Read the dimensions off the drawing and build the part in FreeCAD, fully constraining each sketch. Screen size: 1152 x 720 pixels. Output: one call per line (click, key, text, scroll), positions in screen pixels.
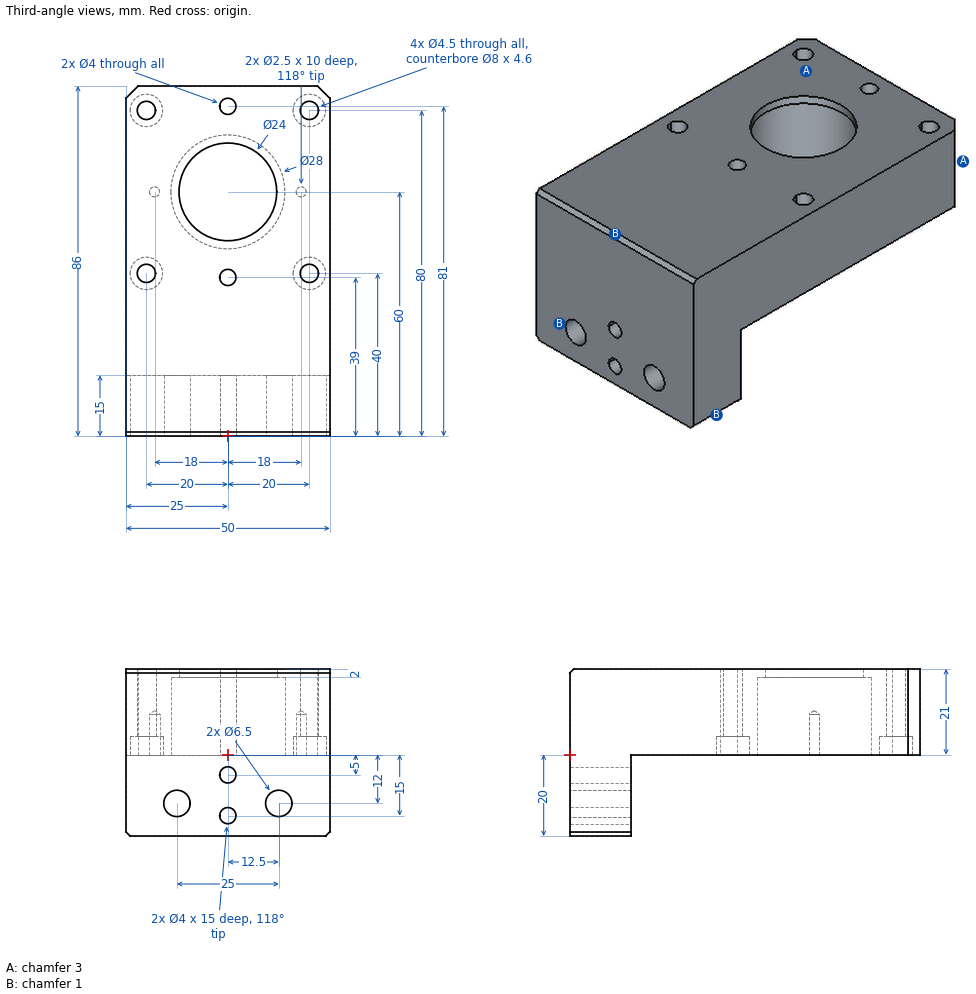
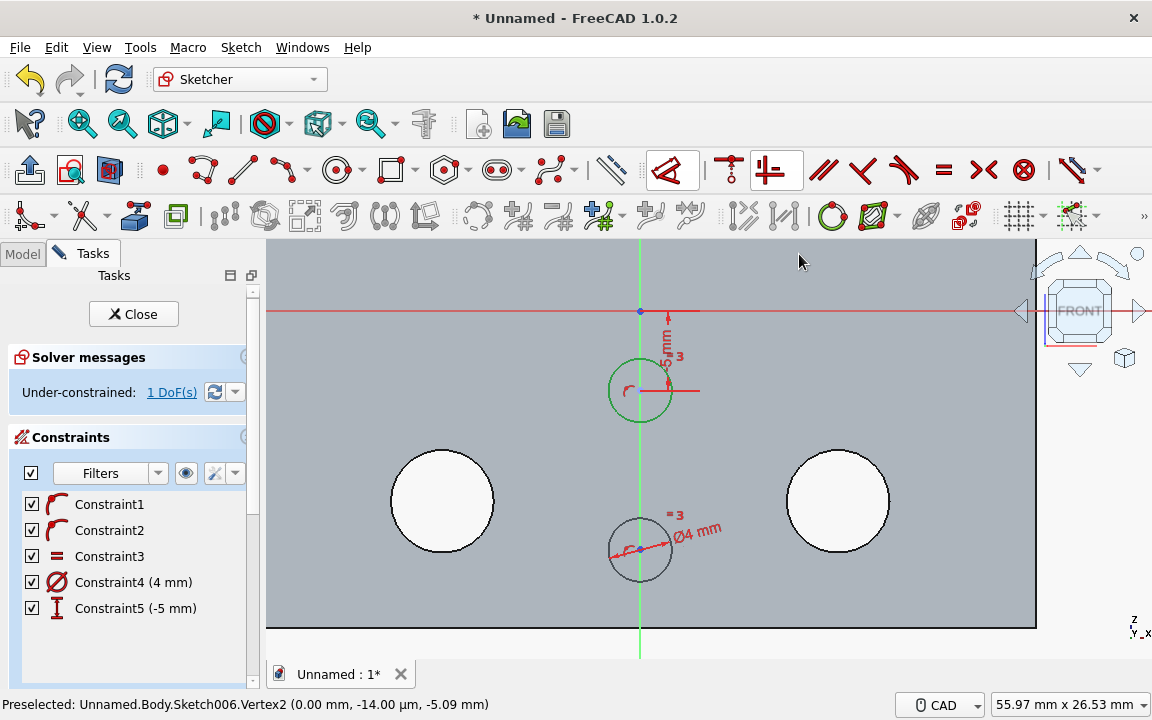
click(640, 550)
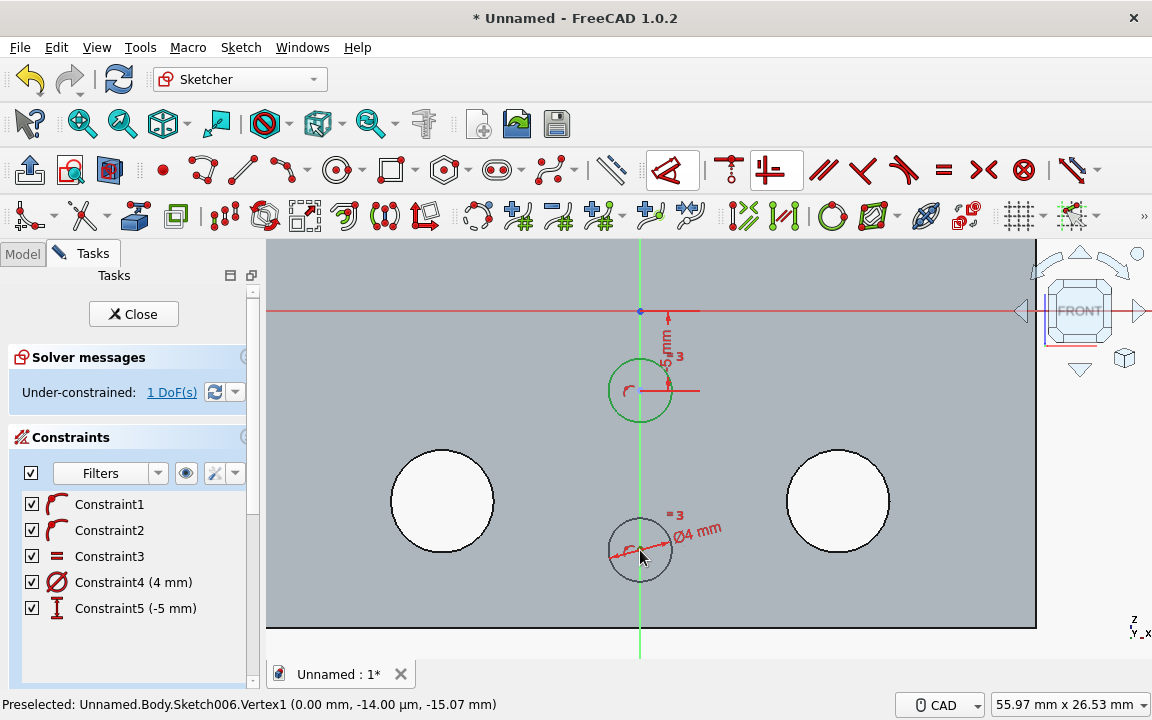
key(i)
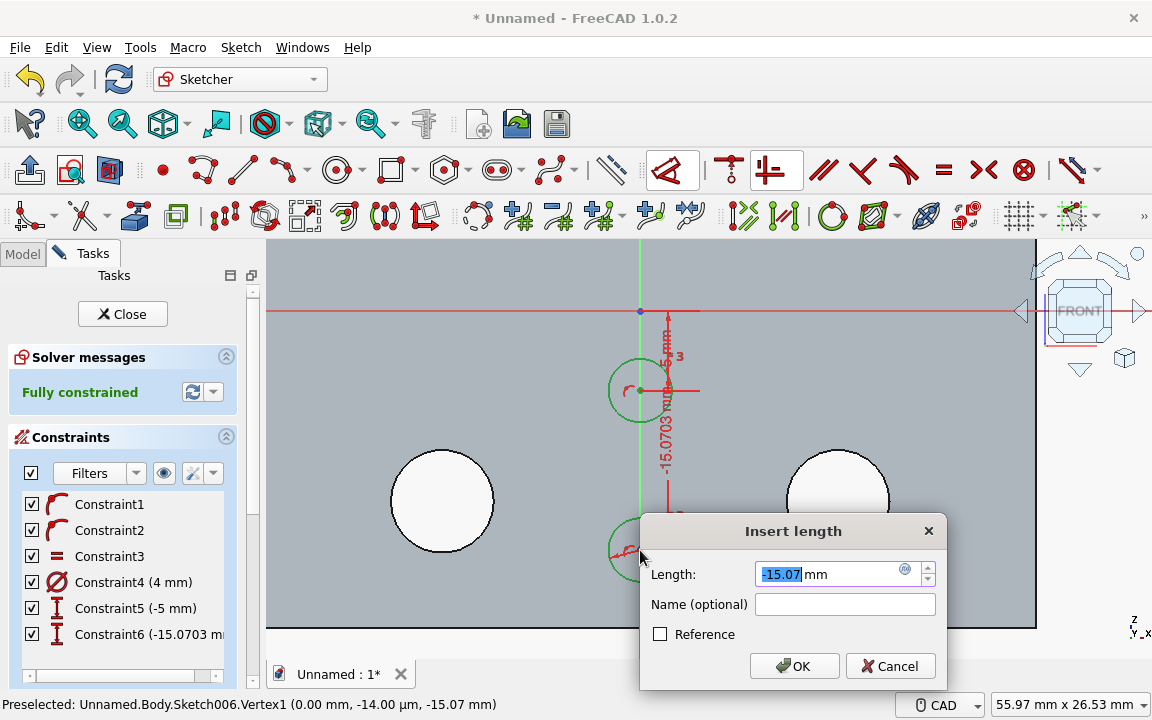
text(-15)
key(Return)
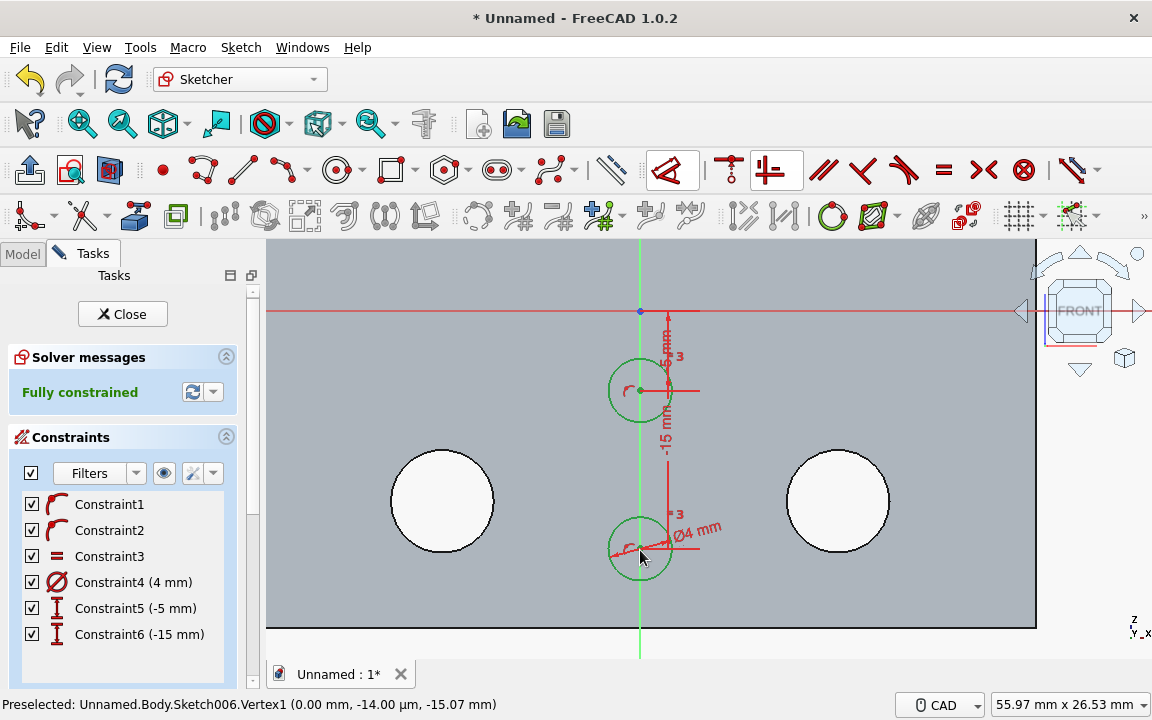
click(123, 314)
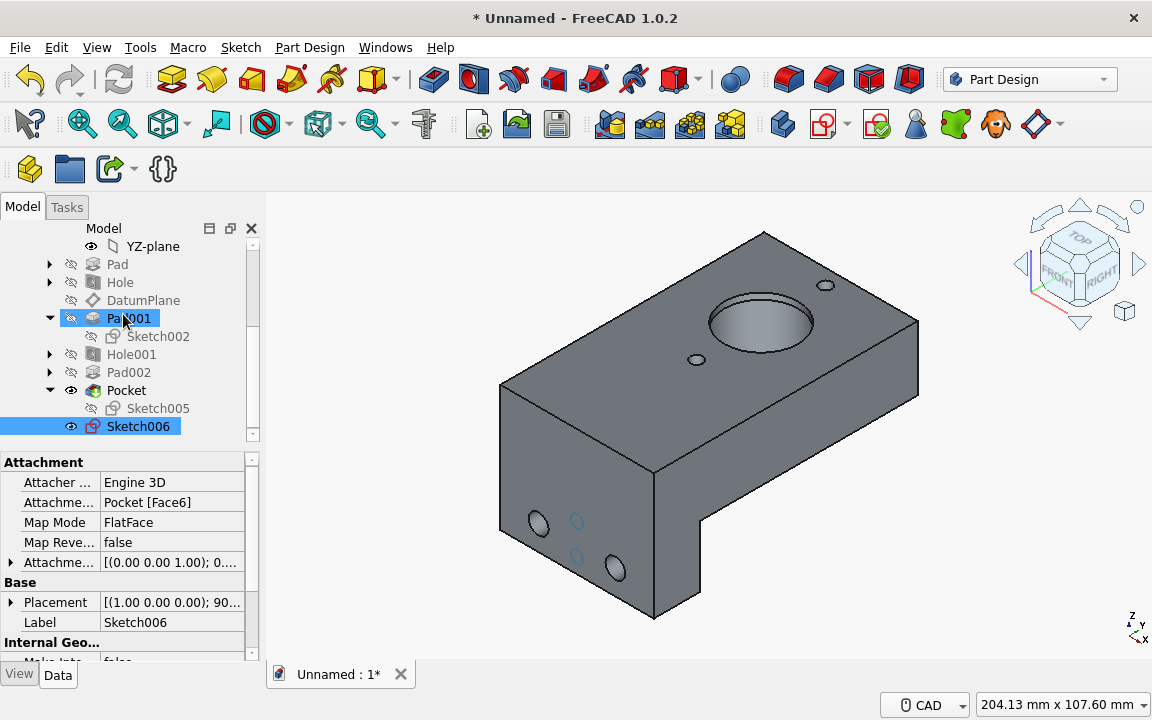
click(474, 80)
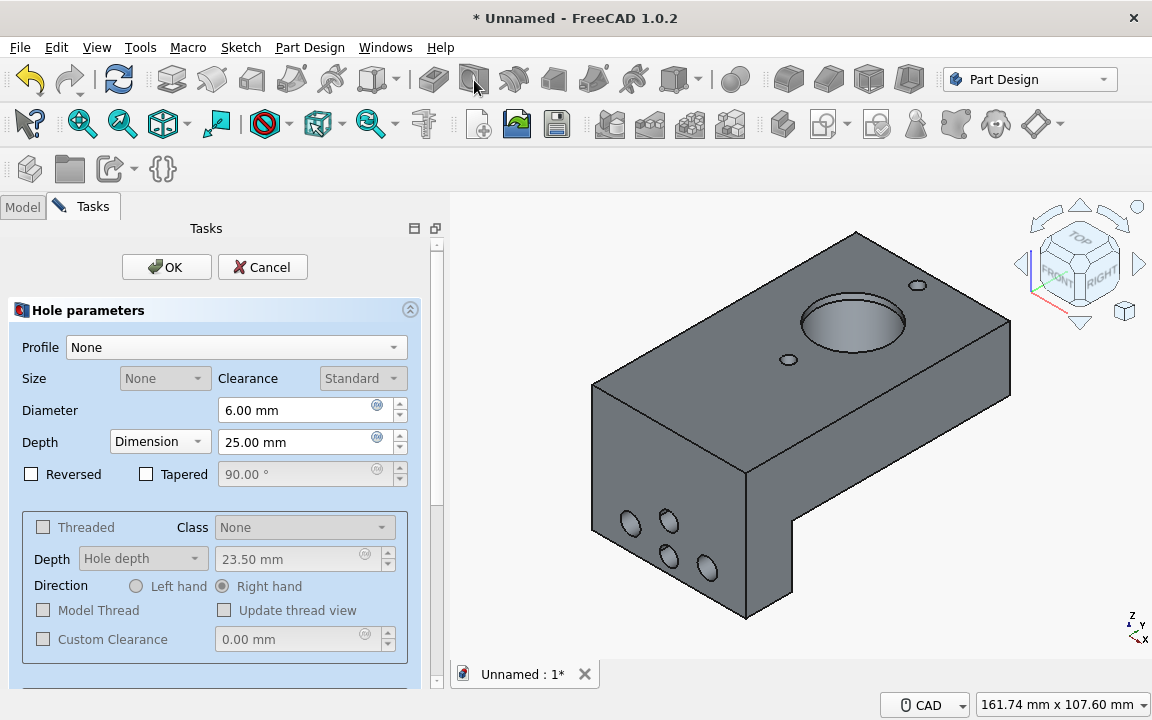
triple_click(305, 410)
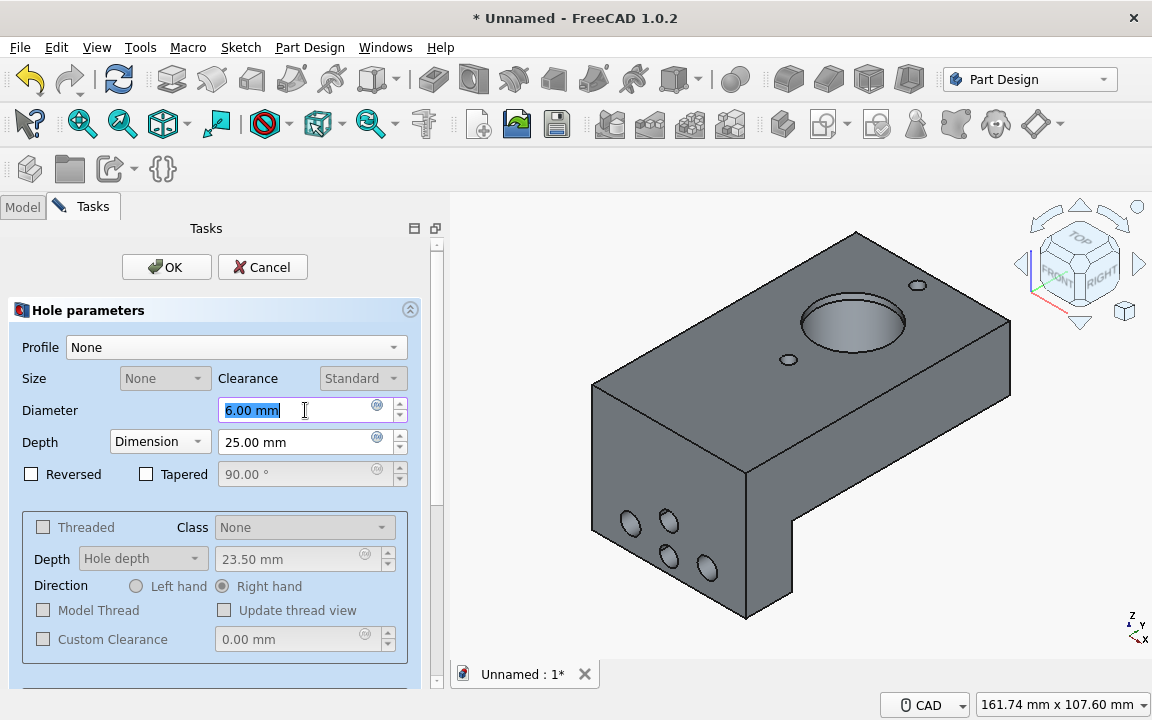
text(4)
key(Tab)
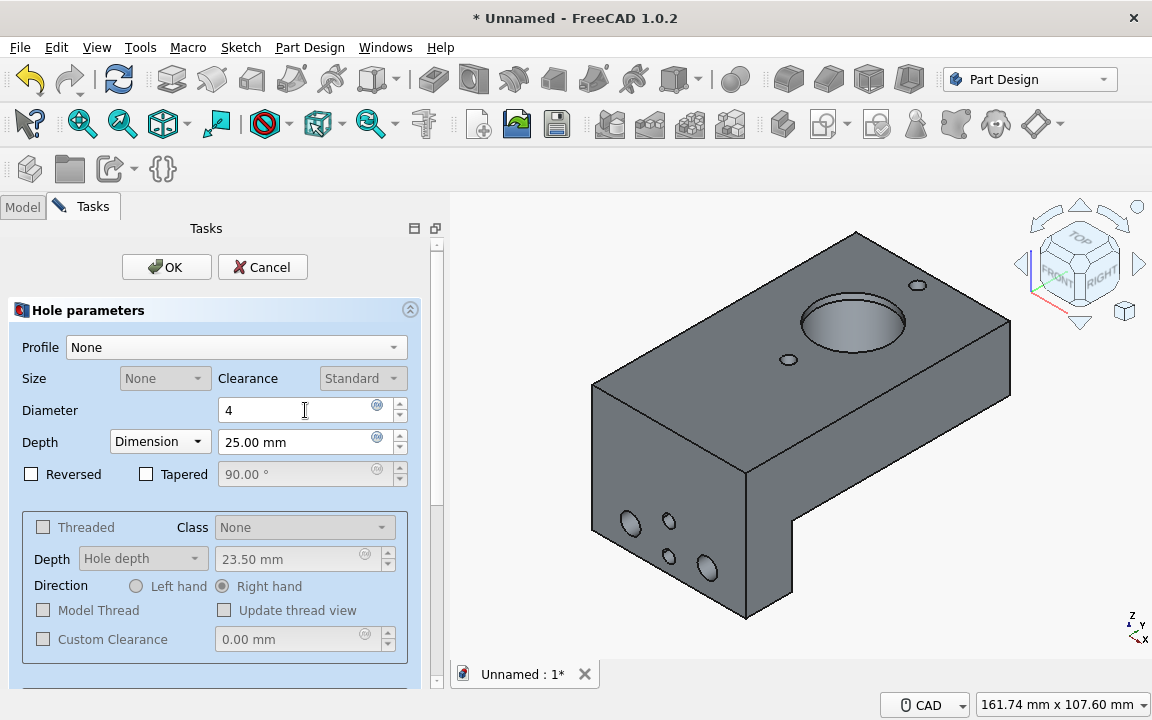
triple_click(305, 442)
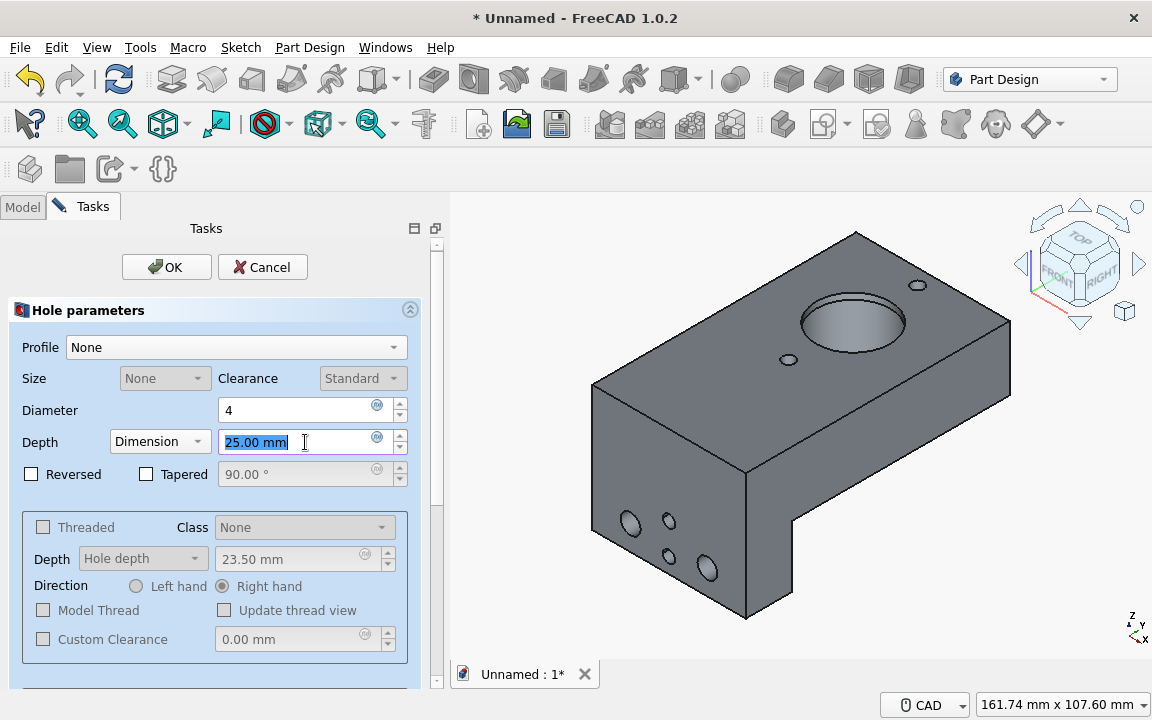
text(15)
key(Tab)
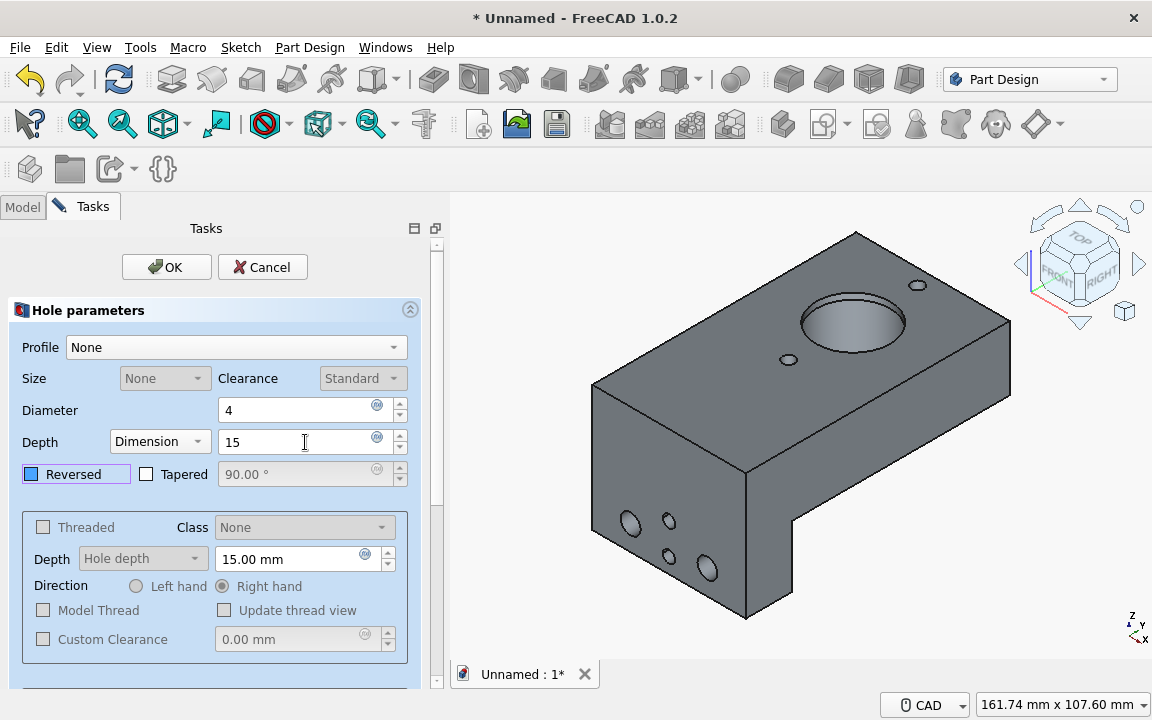
click(167, 267)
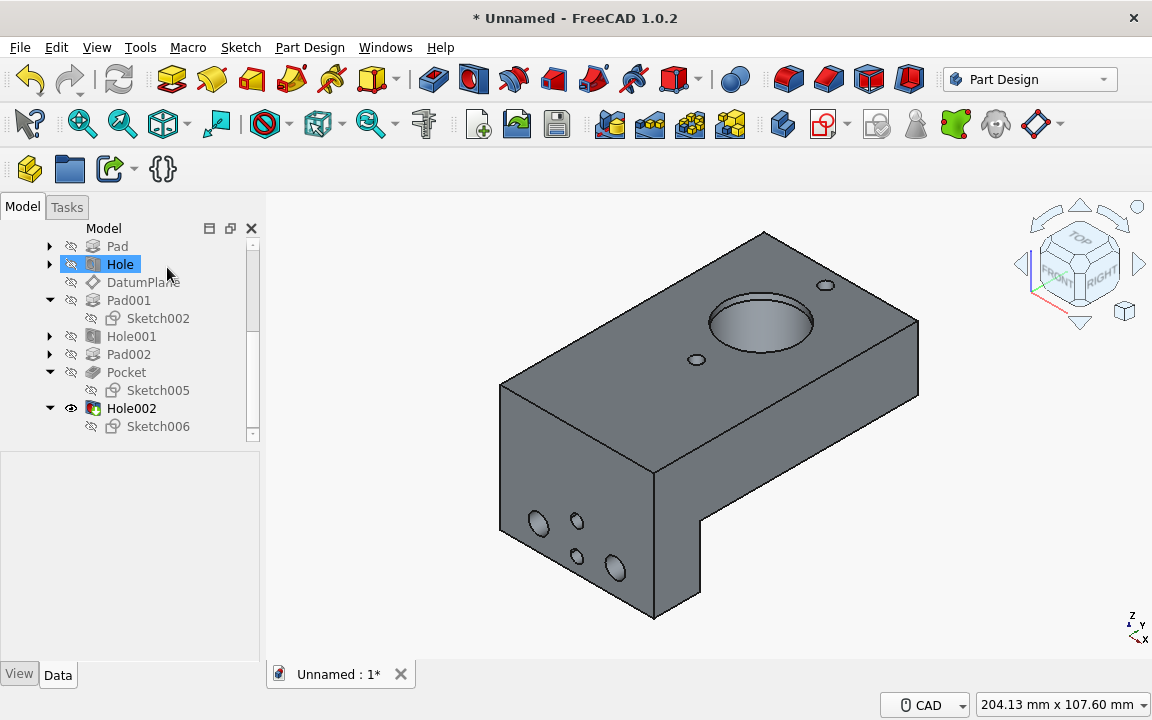
click(824, 124)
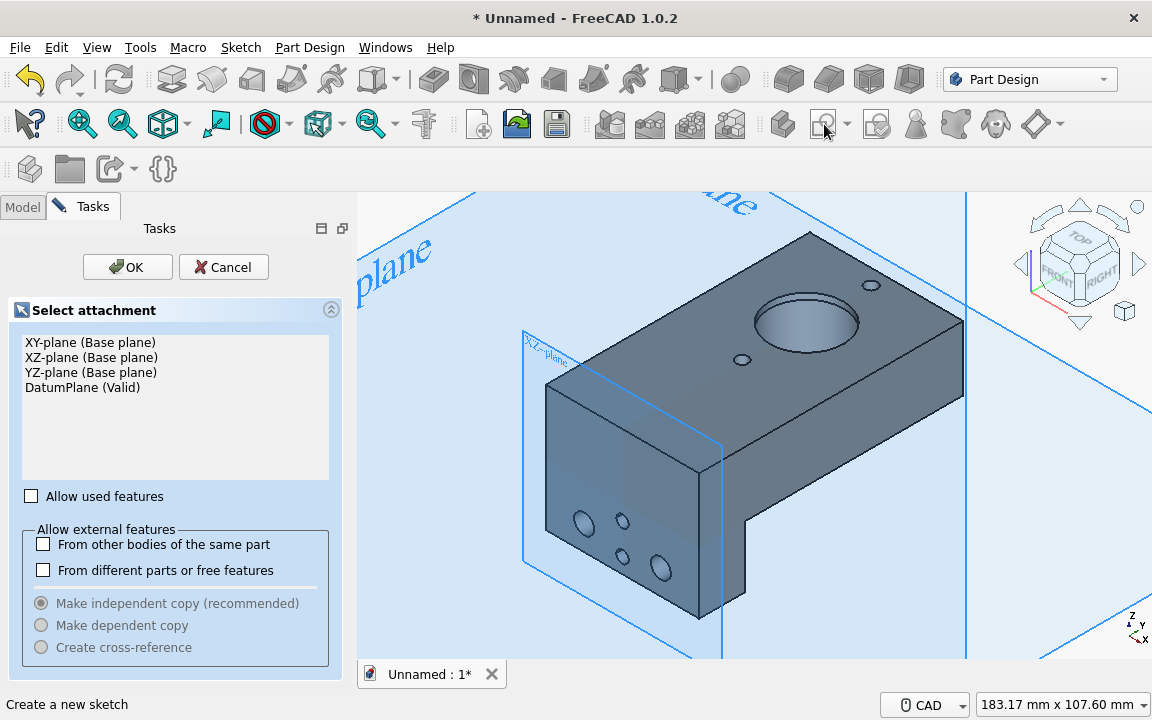
click(82, 342)